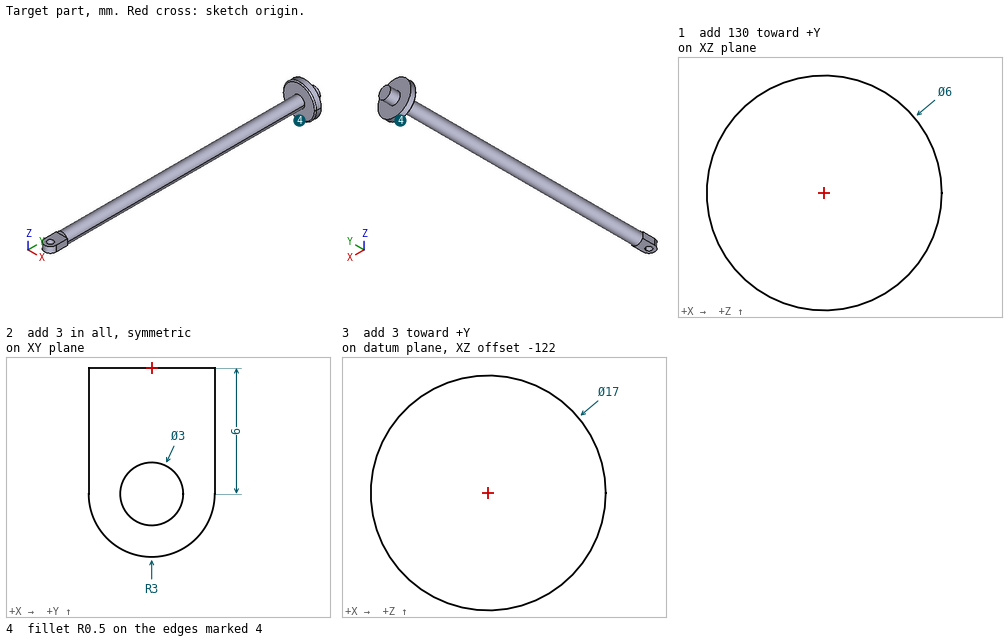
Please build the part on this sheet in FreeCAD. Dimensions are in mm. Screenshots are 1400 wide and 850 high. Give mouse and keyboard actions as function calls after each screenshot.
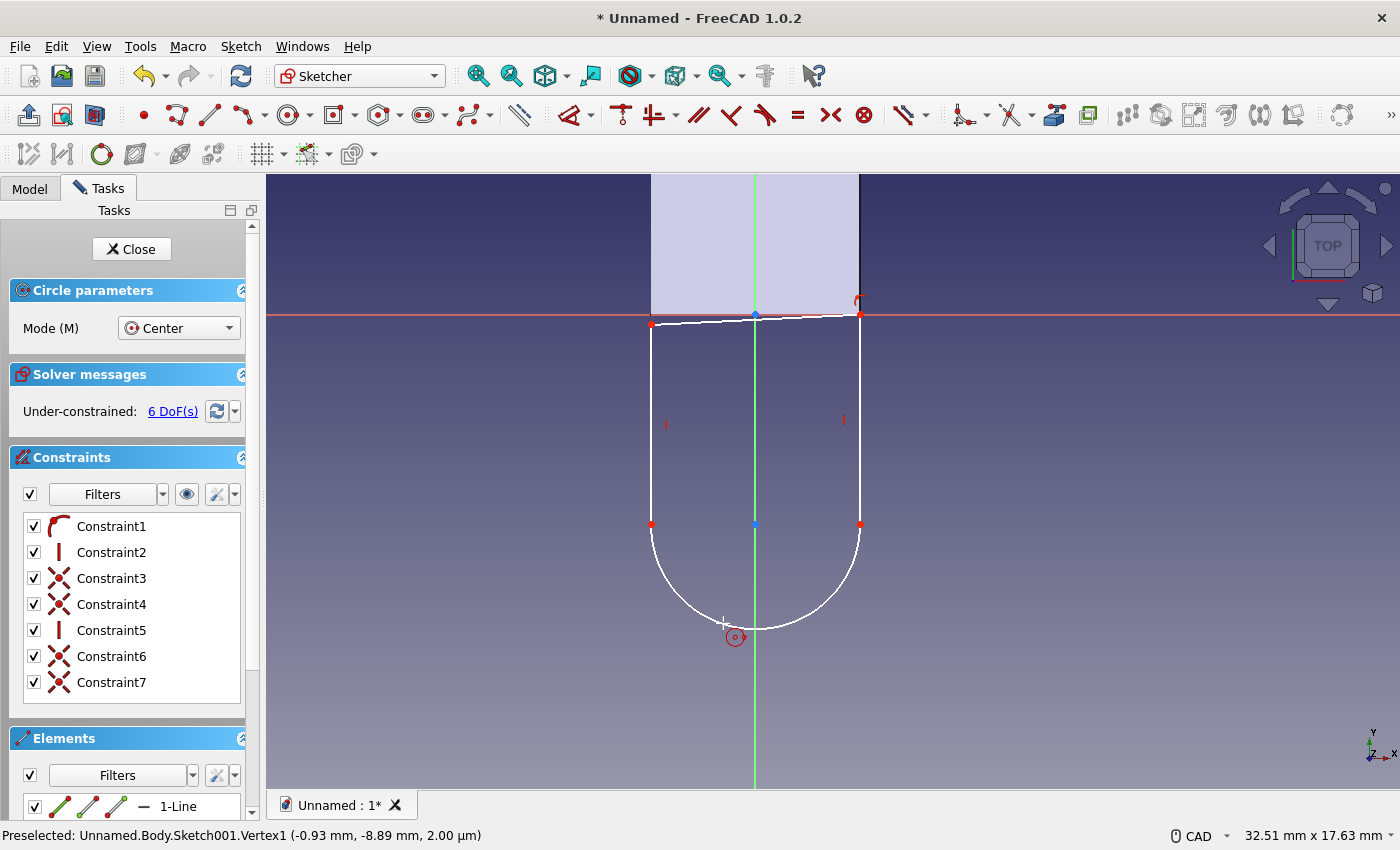
click(755, 524)
click(792, 487)
key(Escape)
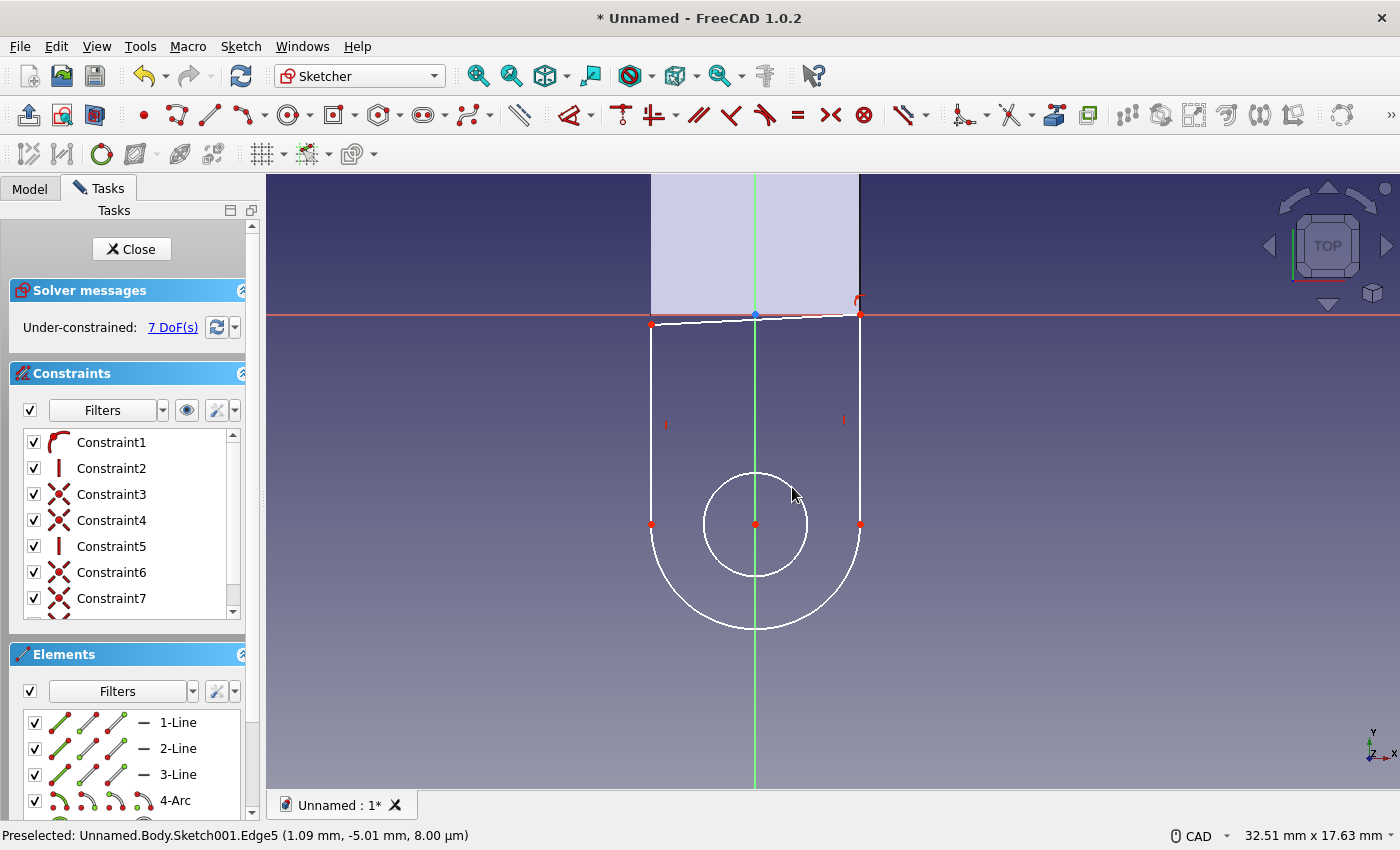
click(860, 462)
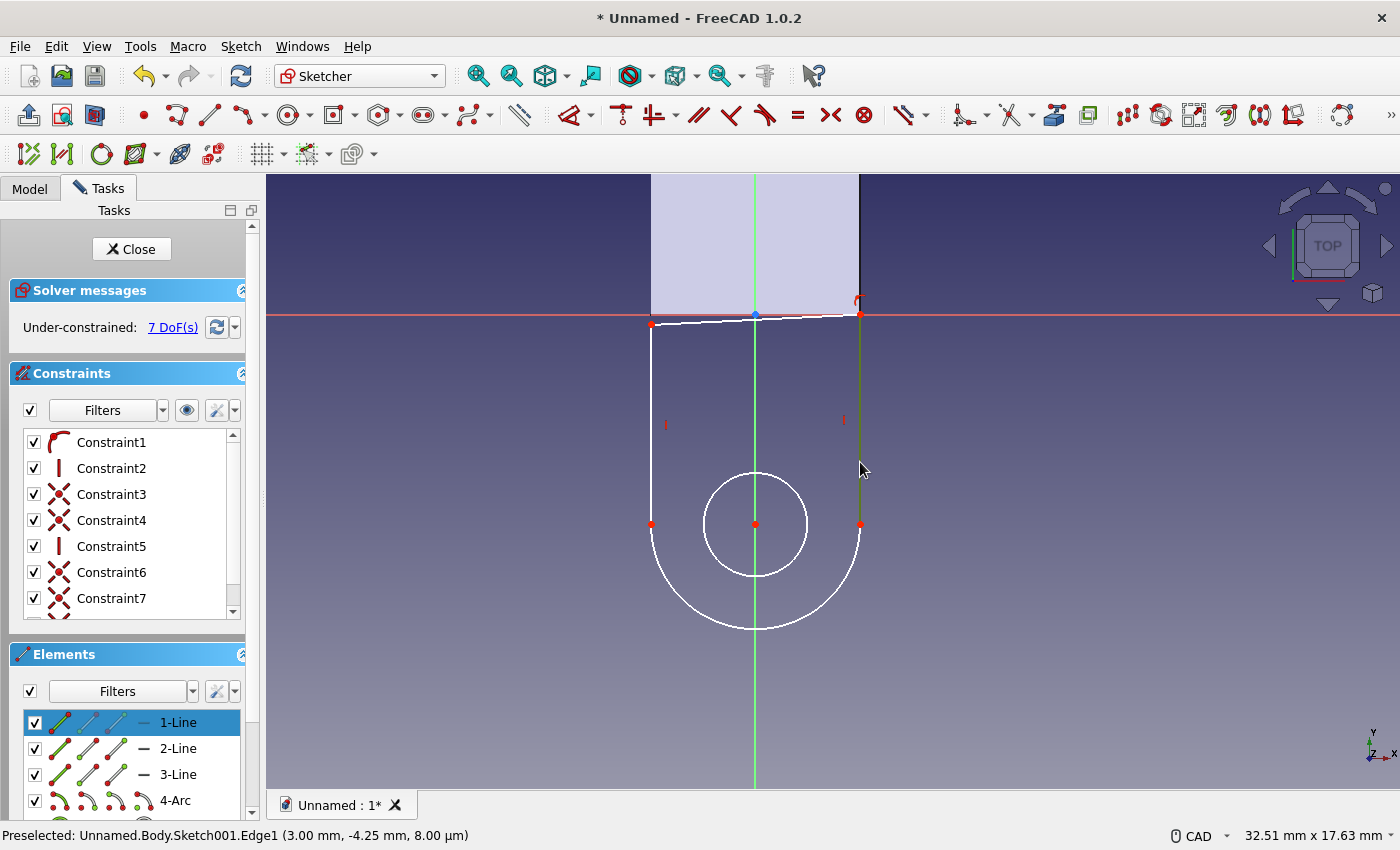
click(694, 609)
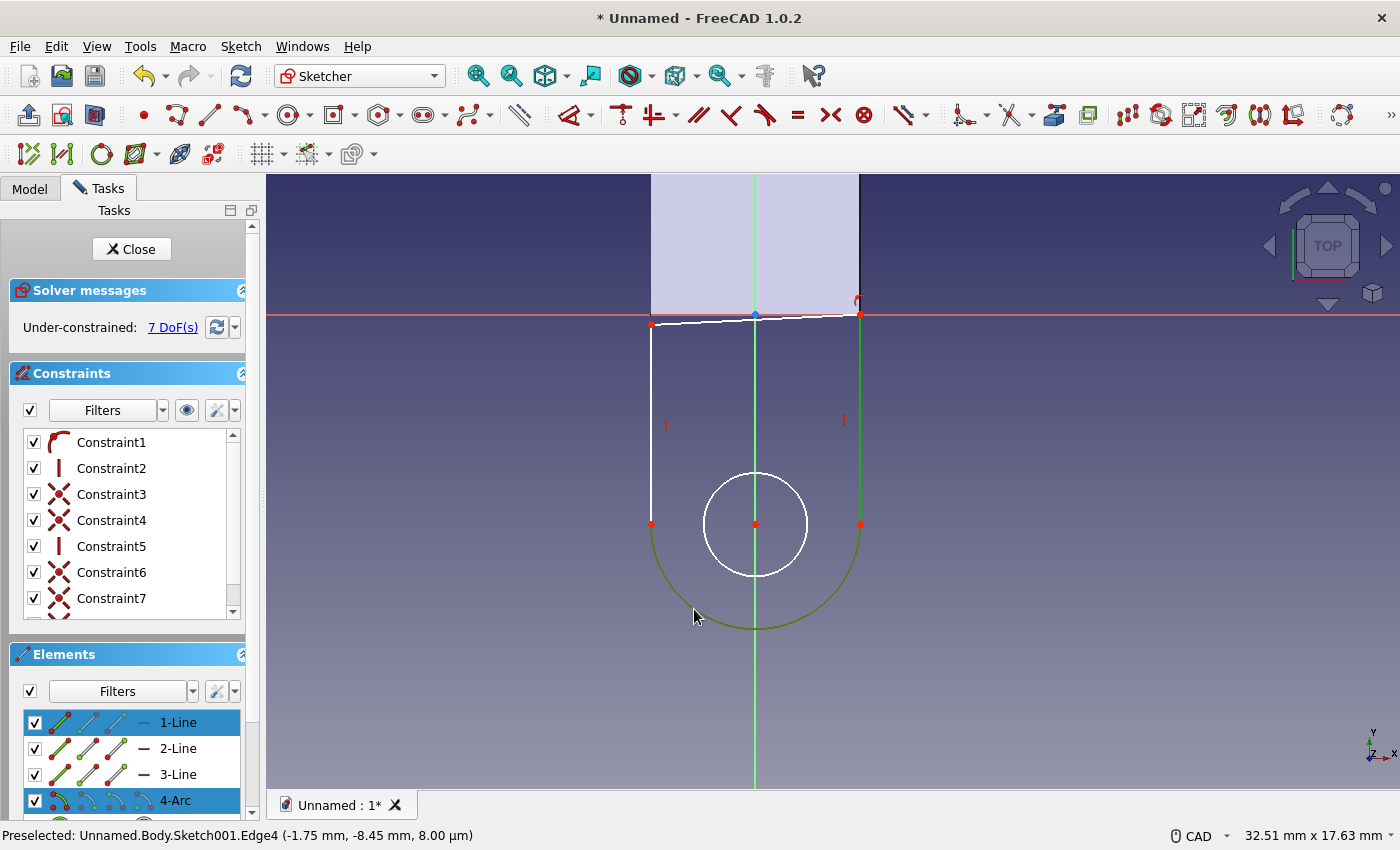
key(t)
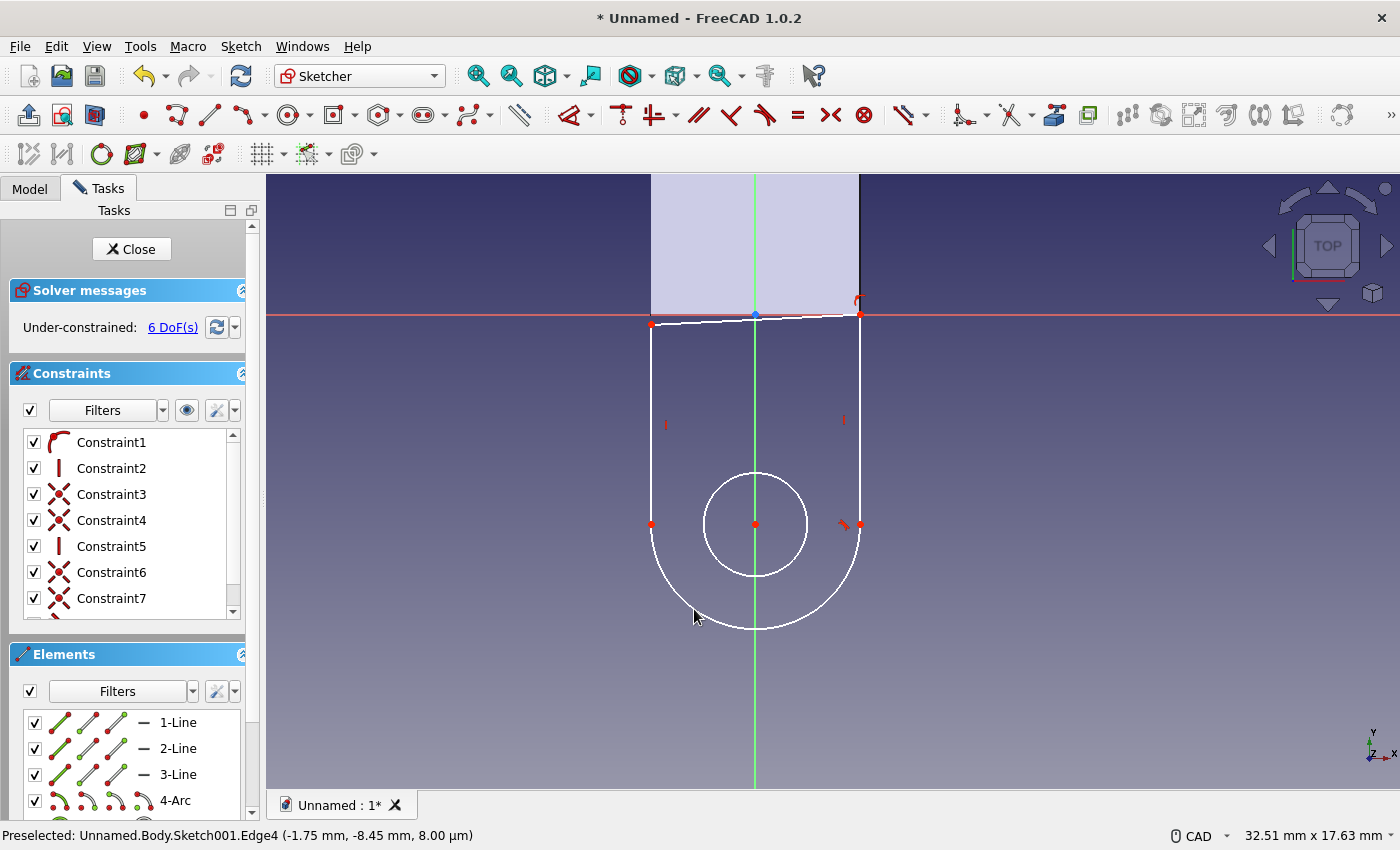
click(651, 385)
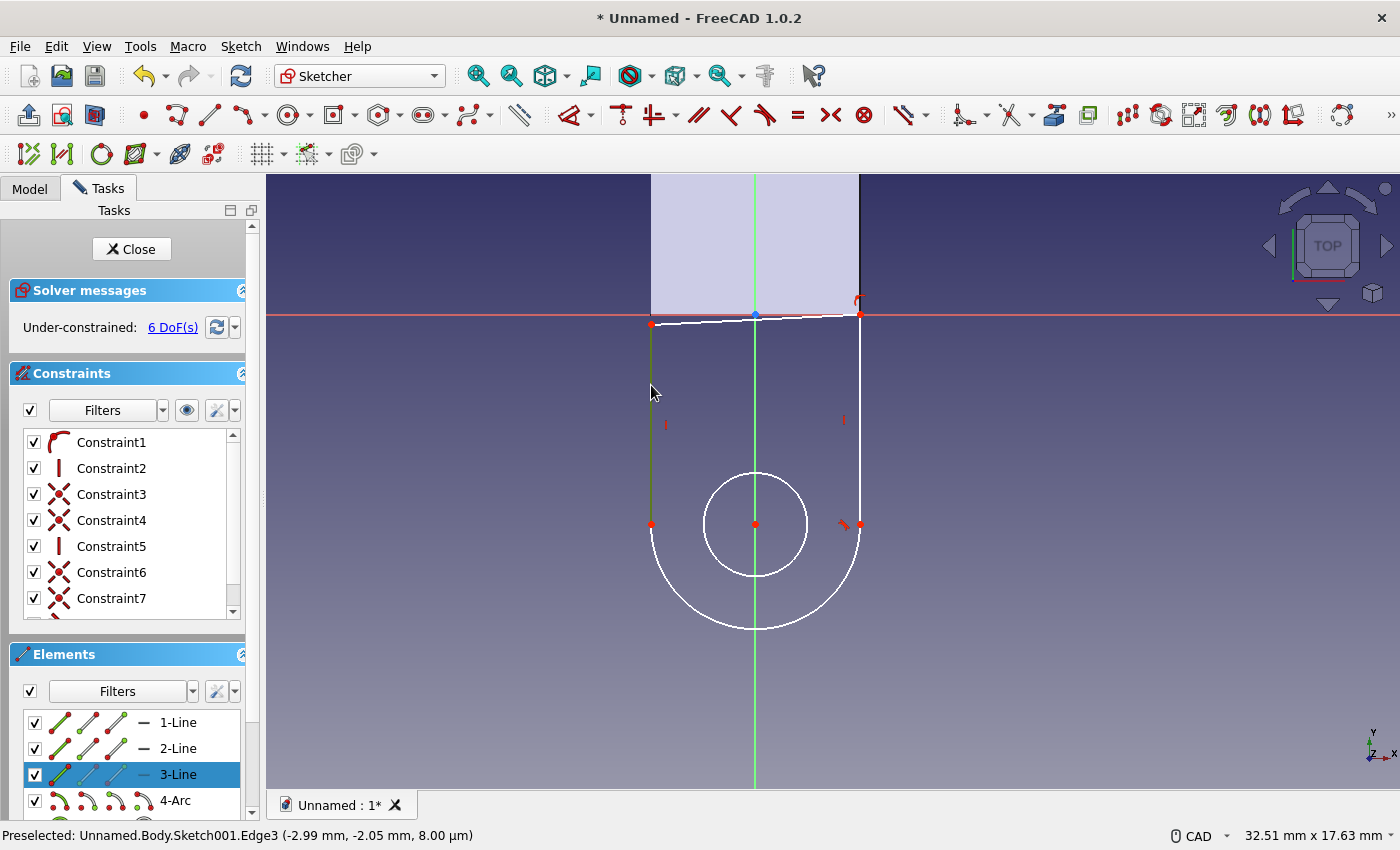
click(694, 609)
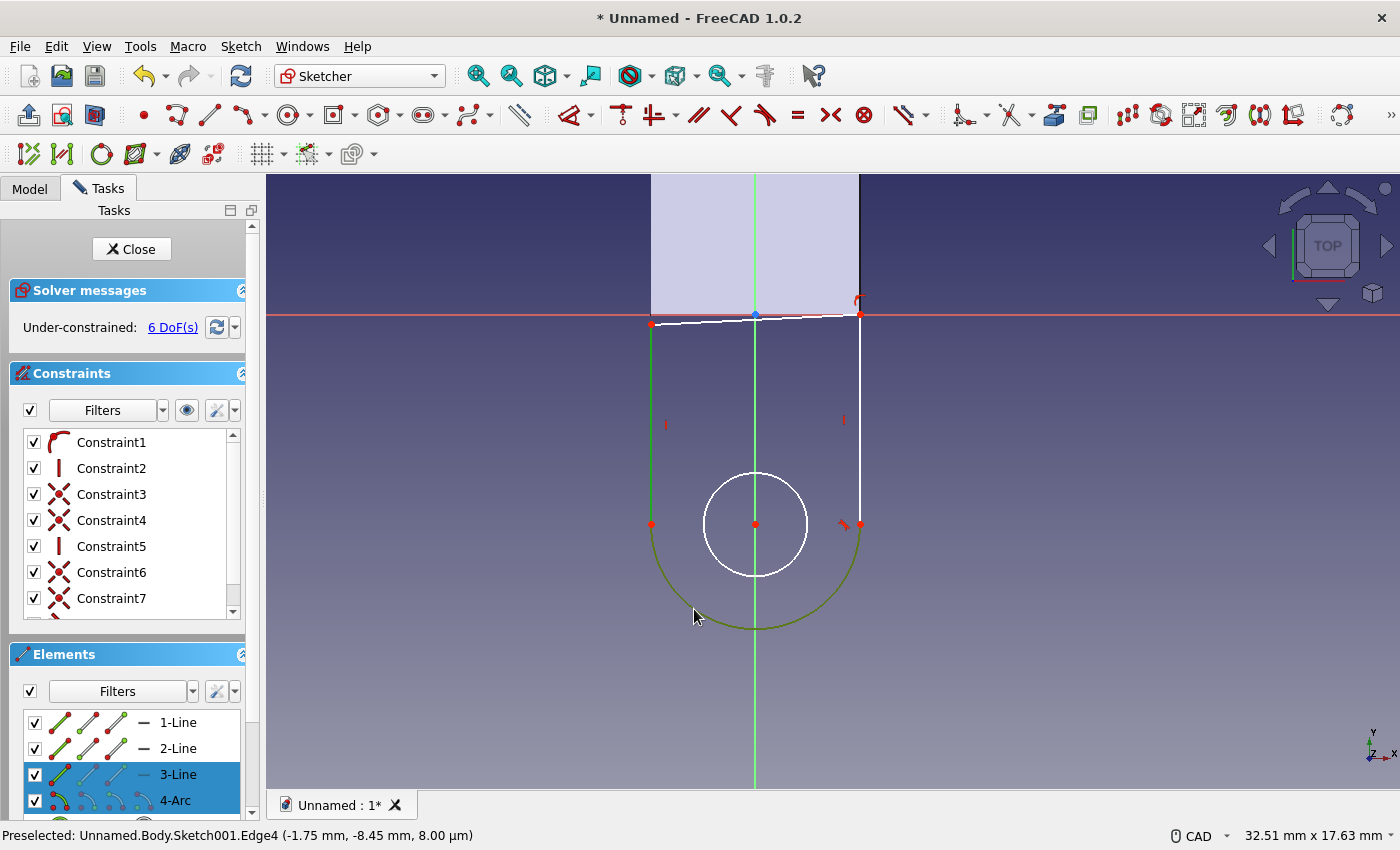
key(t)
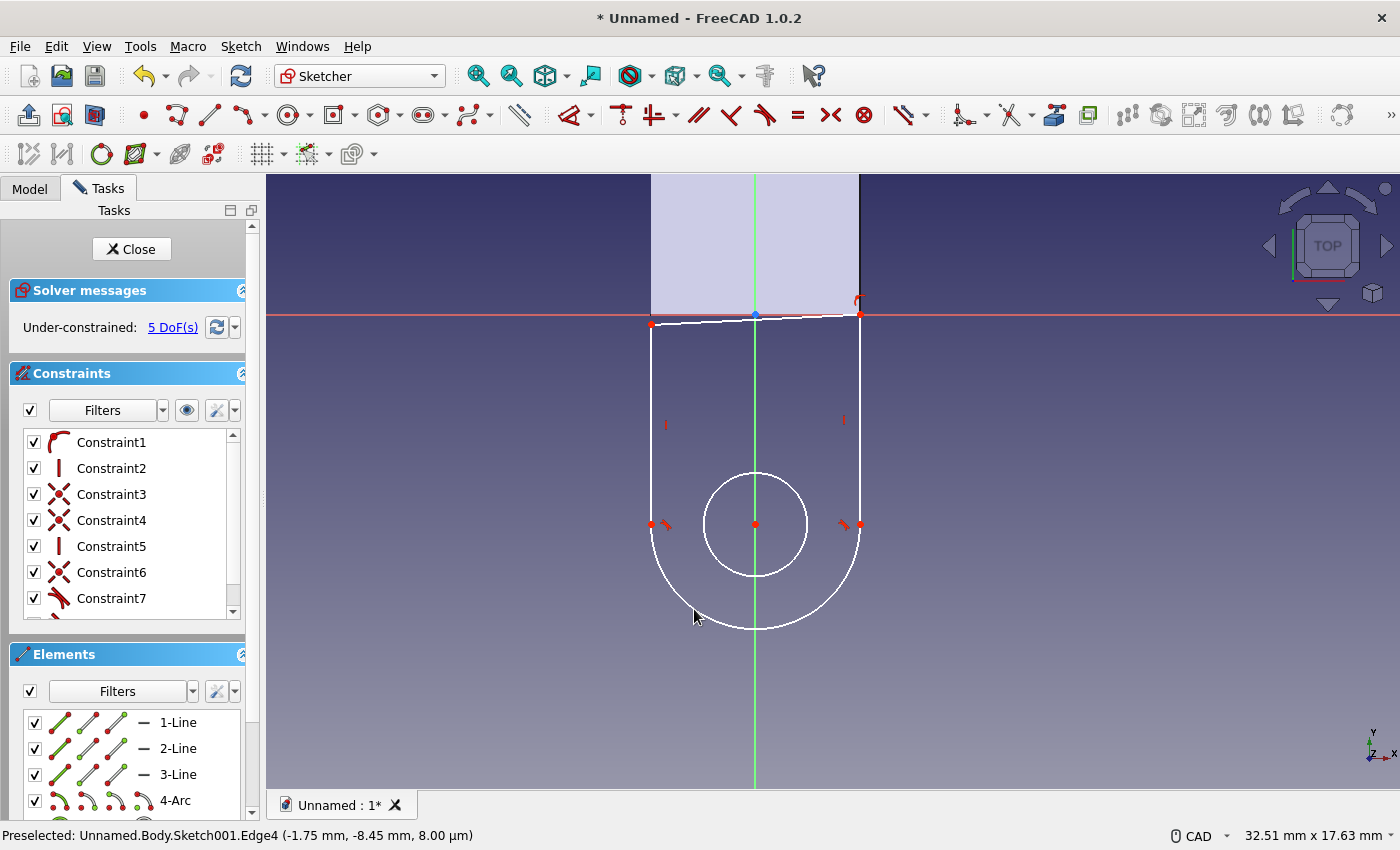
click(797, 318)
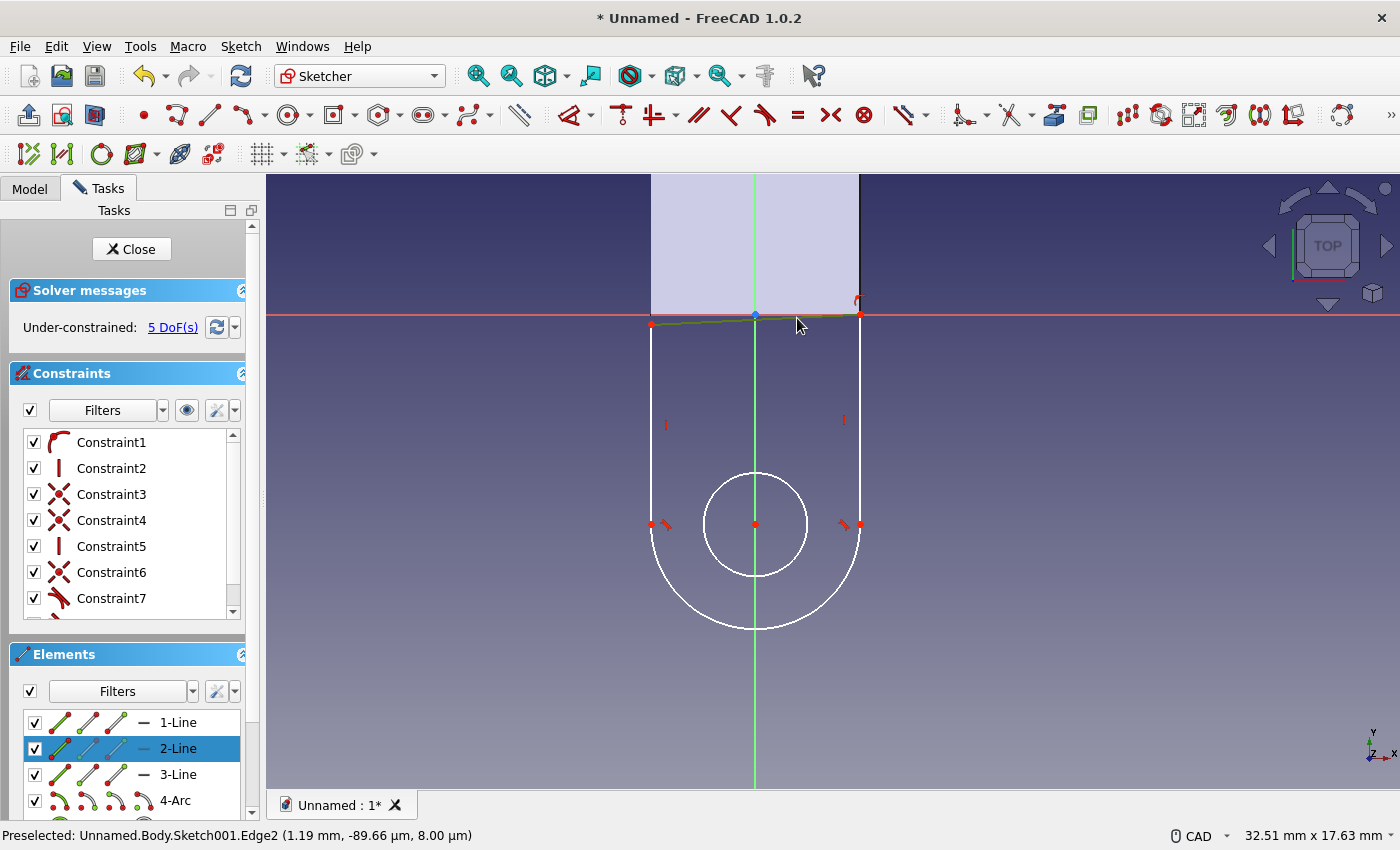
key(h)